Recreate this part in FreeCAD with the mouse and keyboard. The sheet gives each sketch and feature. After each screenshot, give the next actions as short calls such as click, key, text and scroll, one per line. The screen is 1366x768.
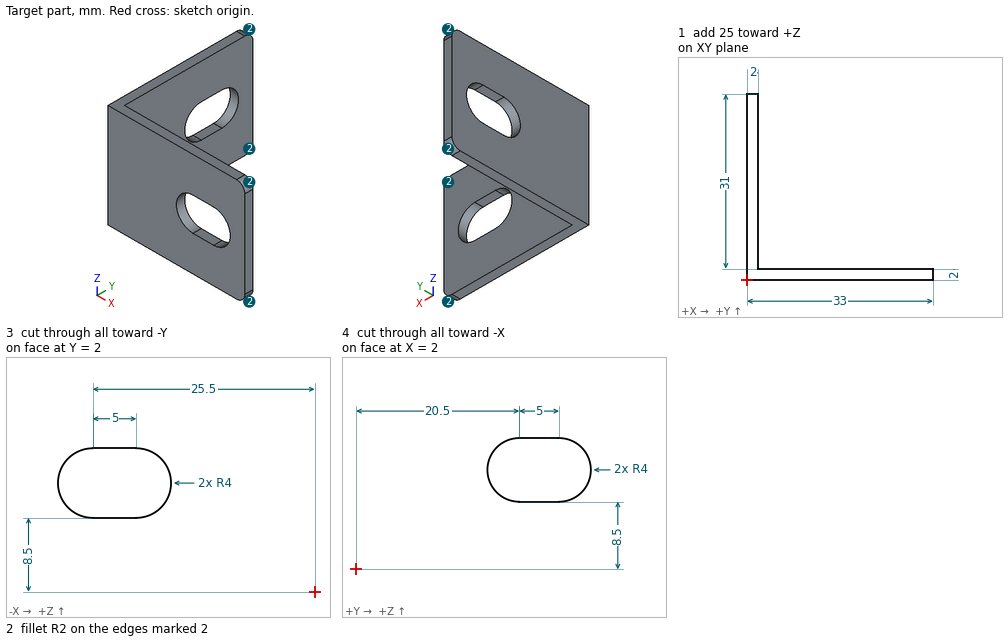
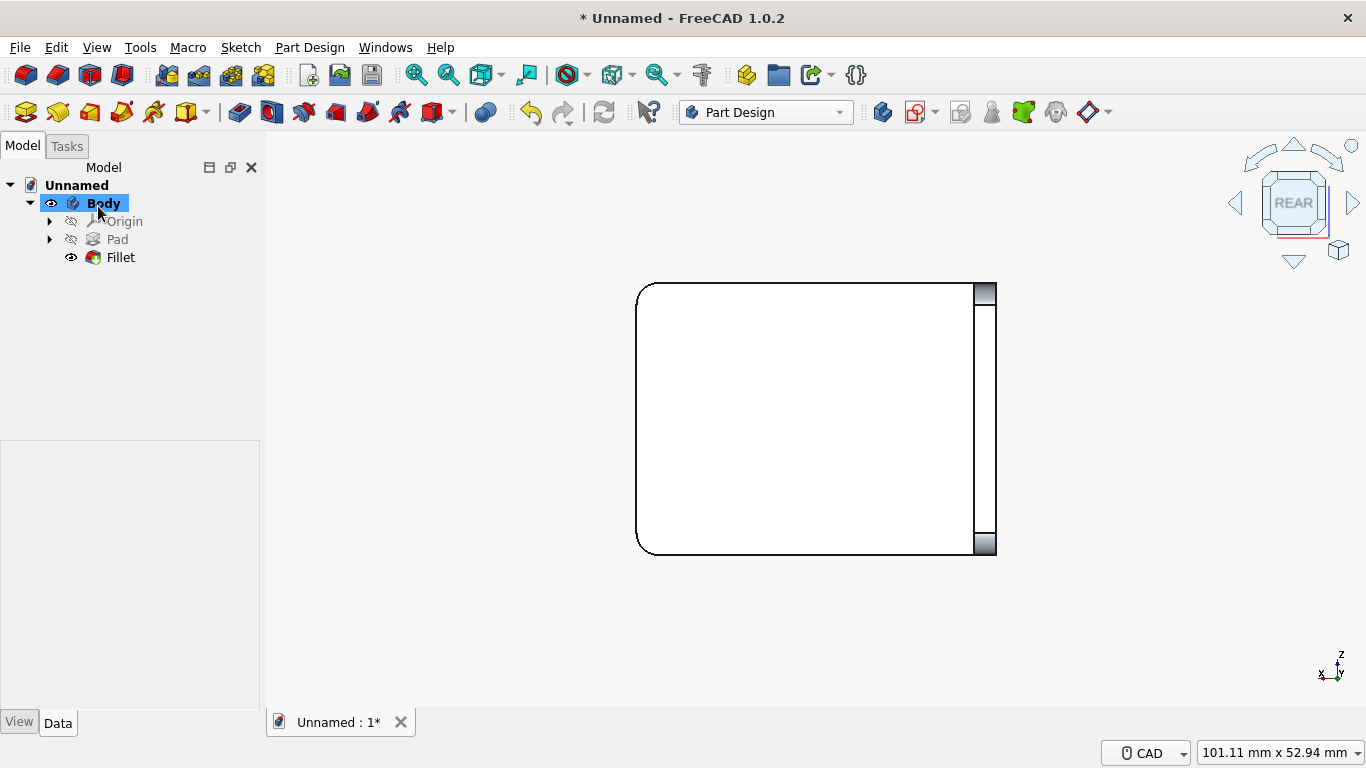
click(805, 418)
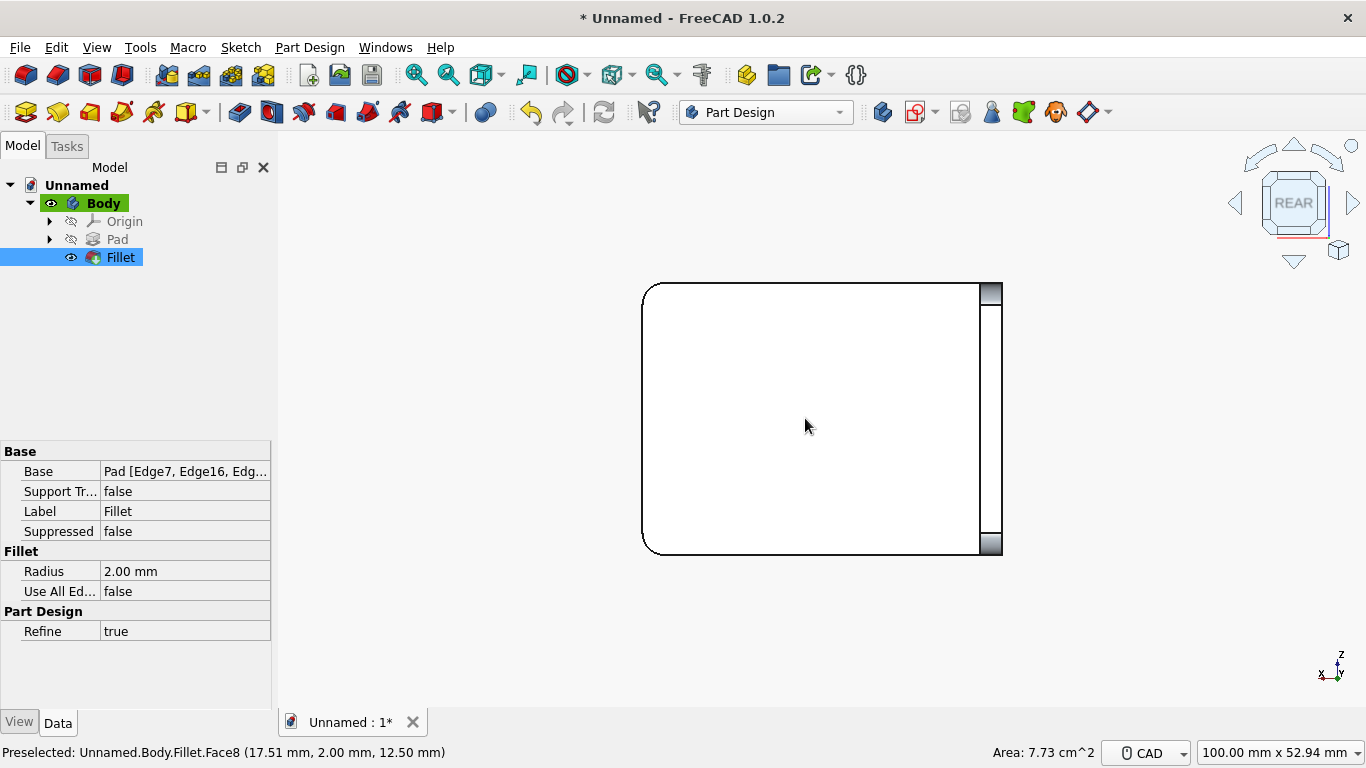
click(916, 112)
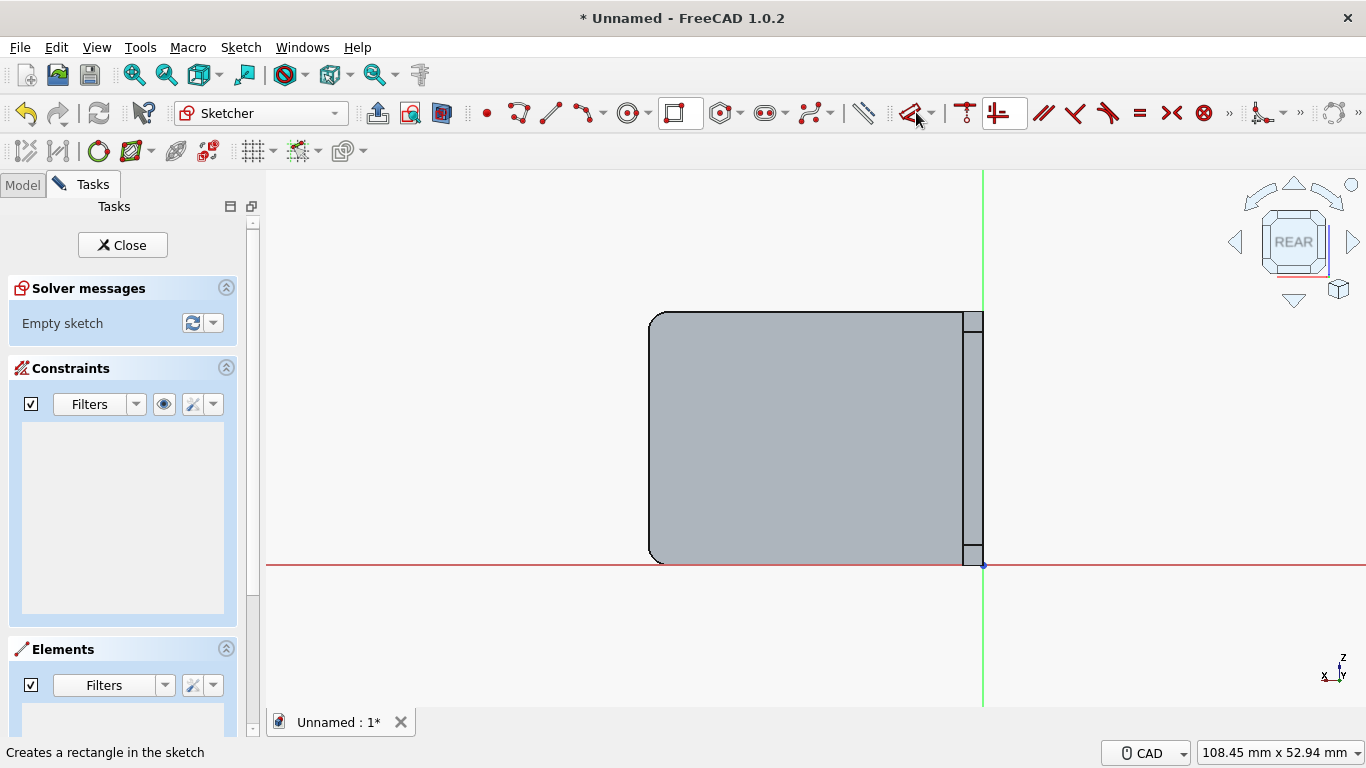
key(q)
key(s)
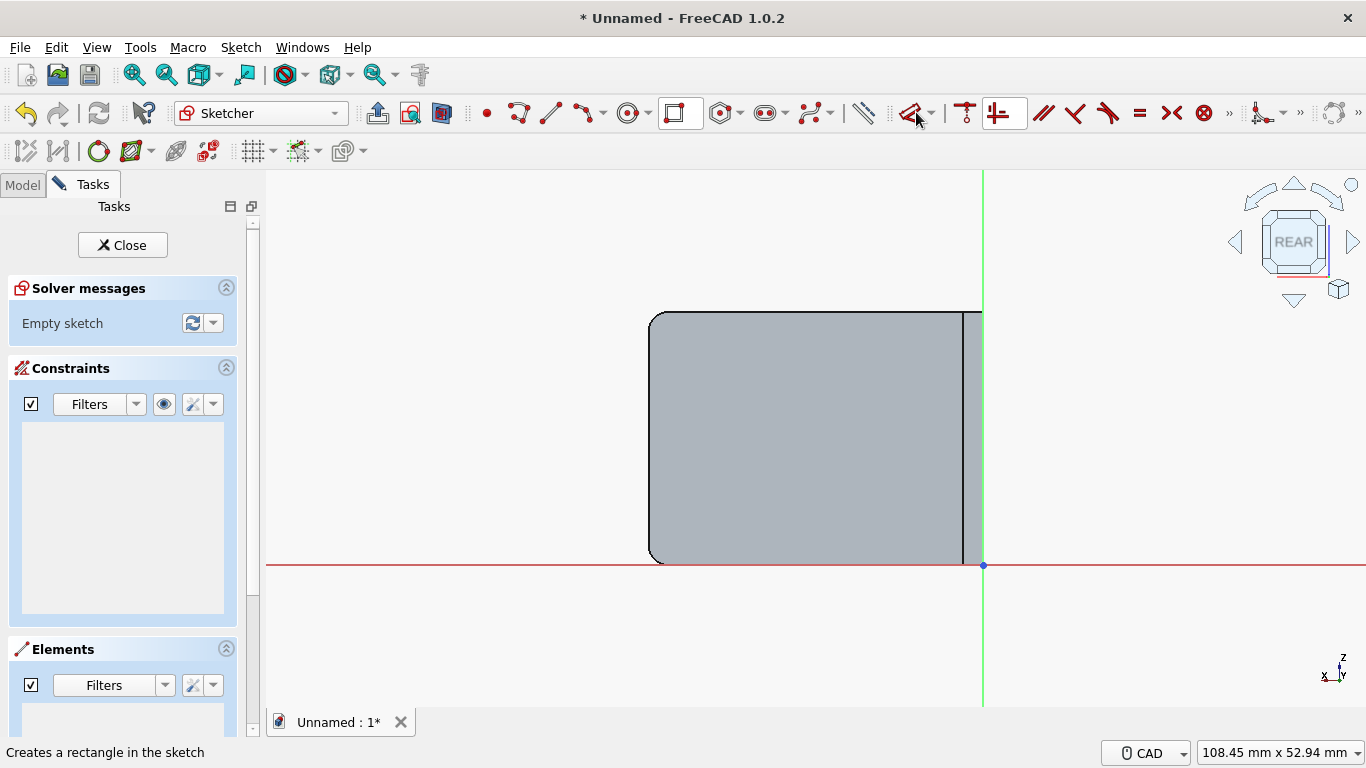
scroll(904, 517, up, 4)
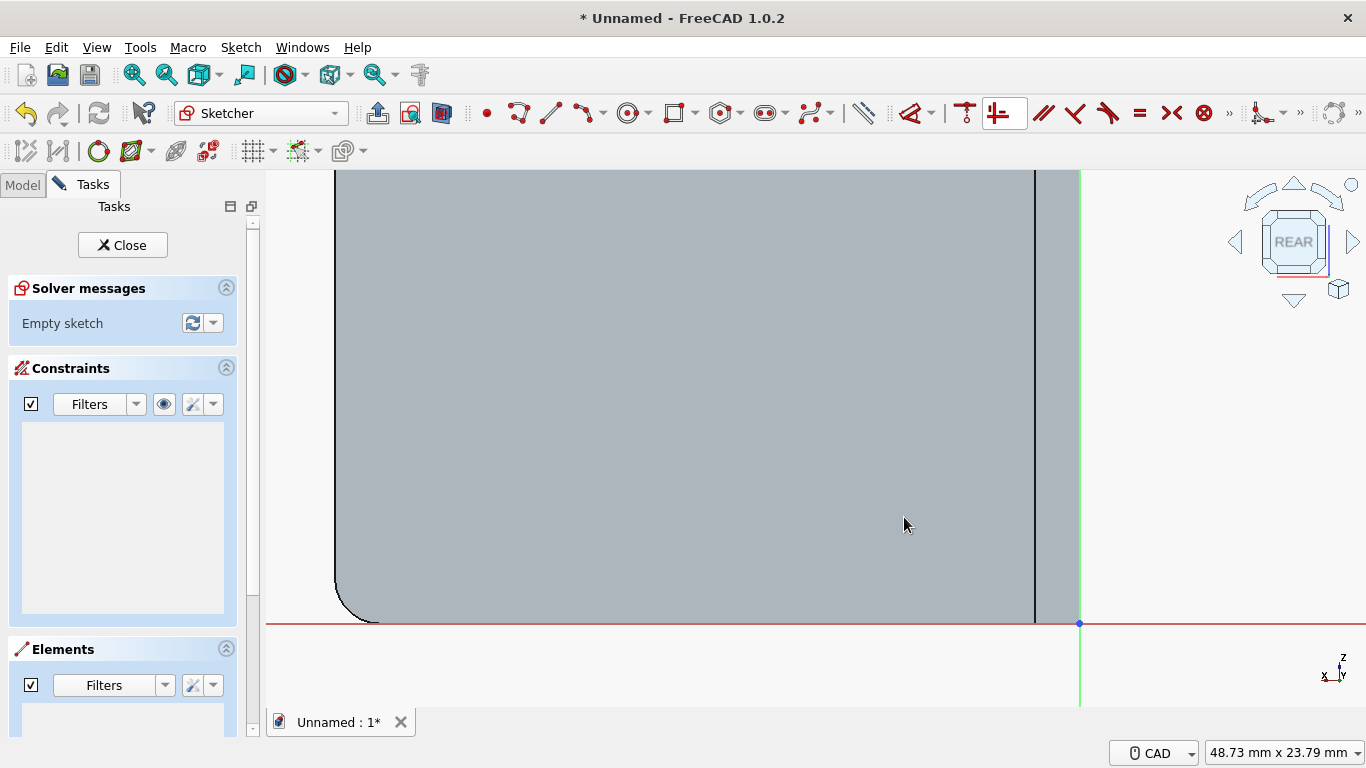
key(g)
key(s)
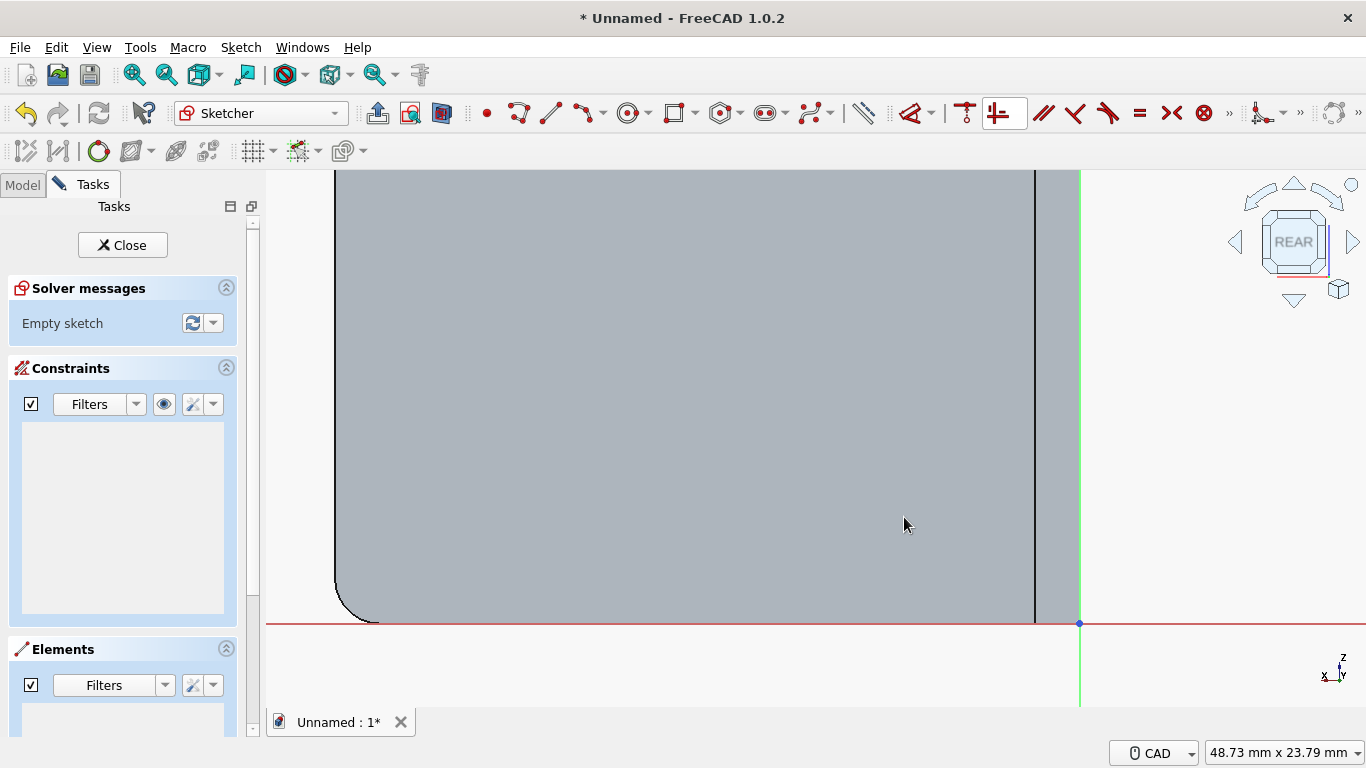
click(504, 342)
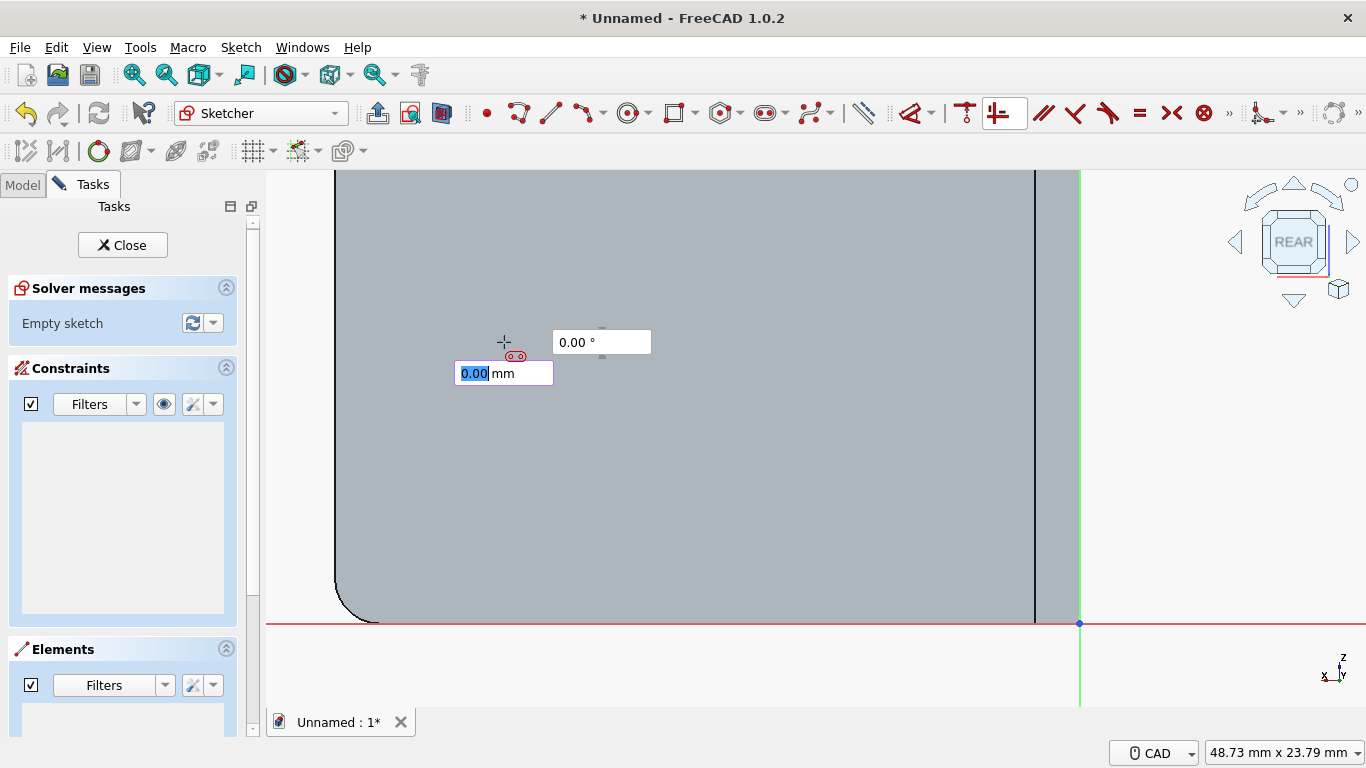
click(617, 342)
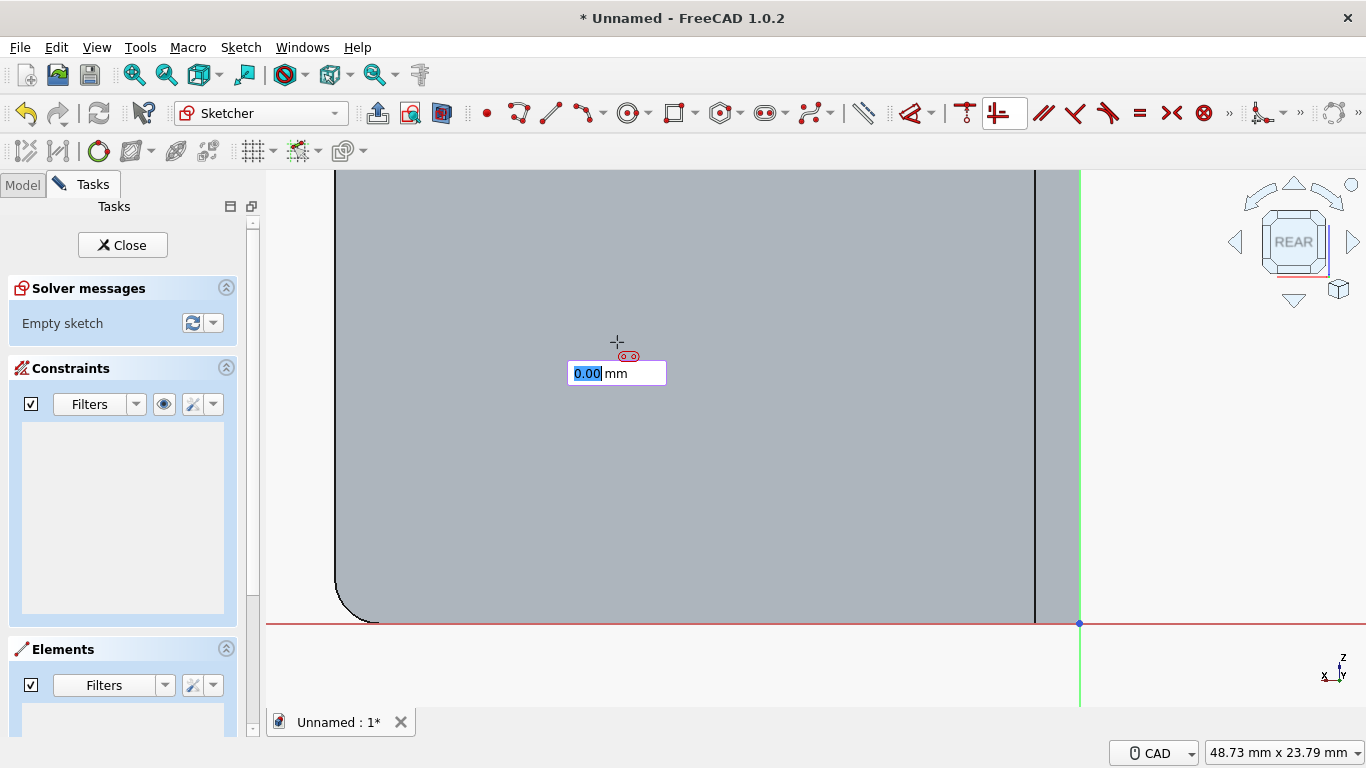
click(561, 432)
key(Escape)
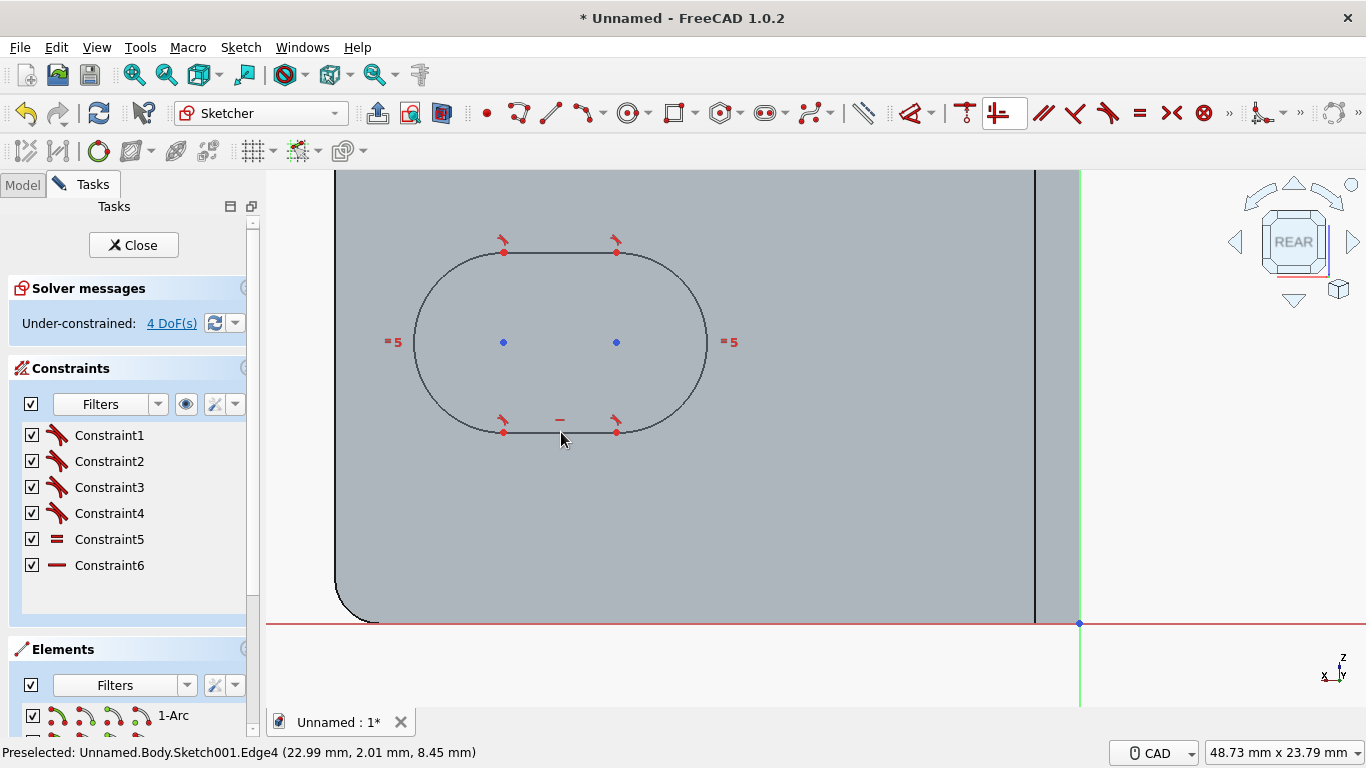
click(431, 290)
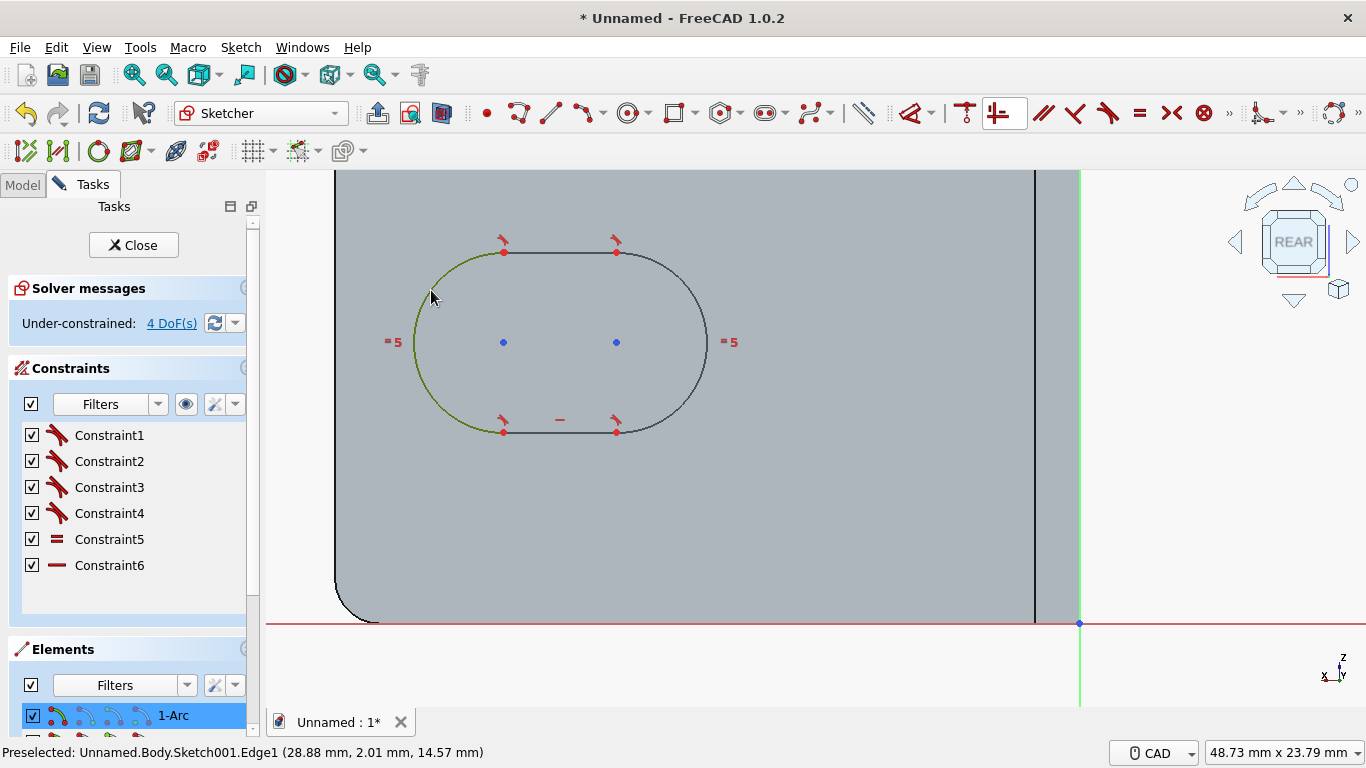
key(k)
key(r)